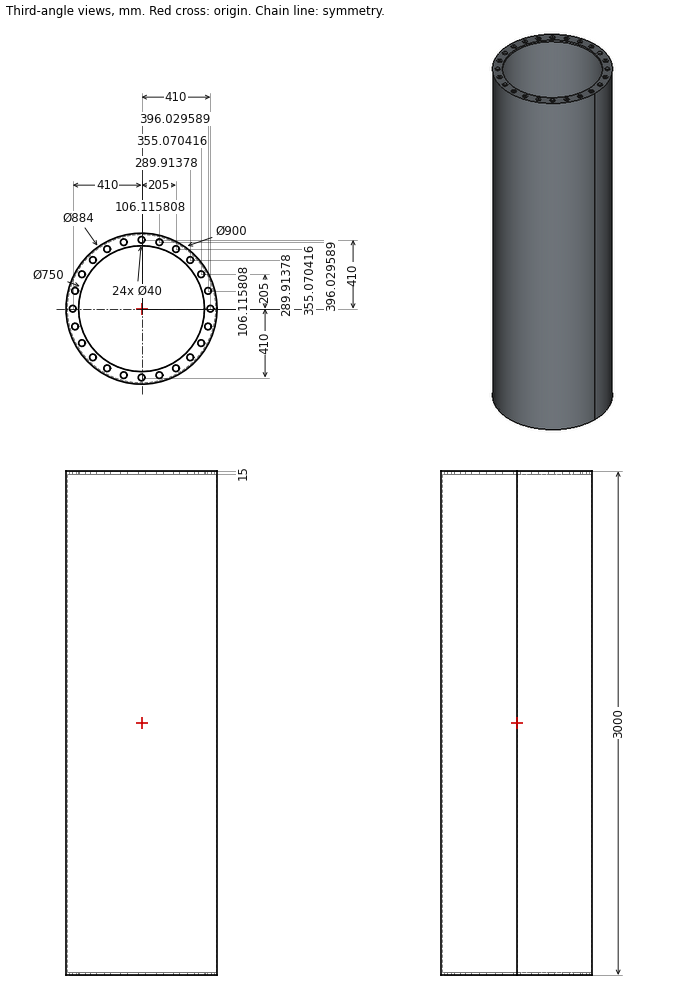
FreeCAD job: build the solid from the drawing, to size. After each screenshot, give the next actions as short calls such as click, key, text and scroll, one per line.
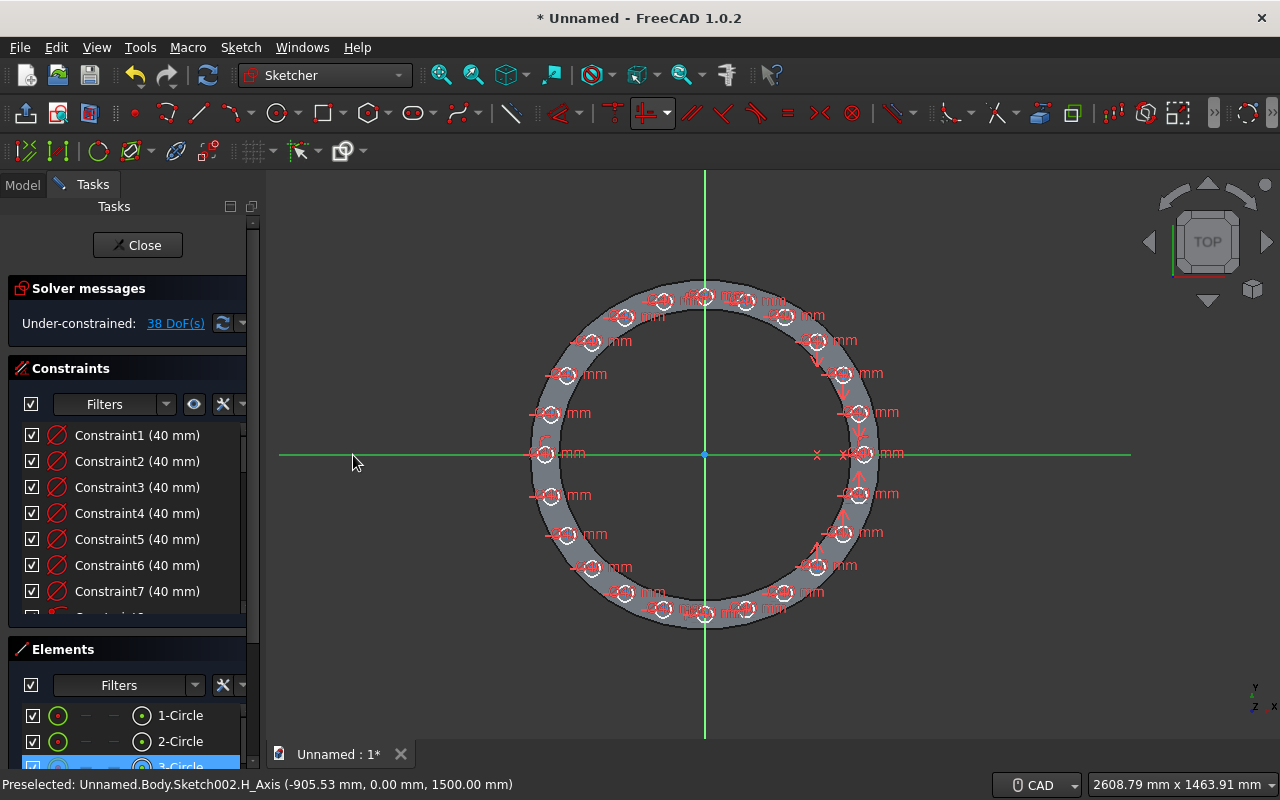
click(820, 114)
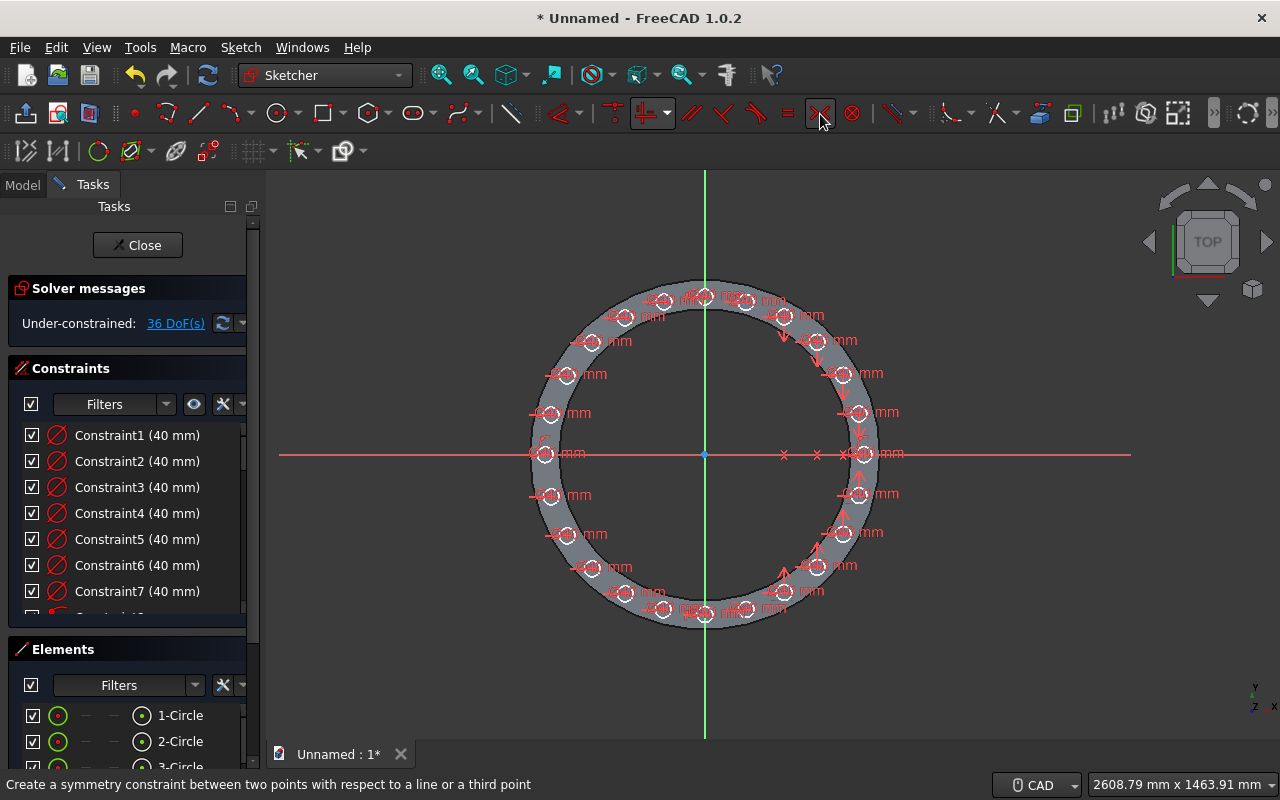
click(746, 302)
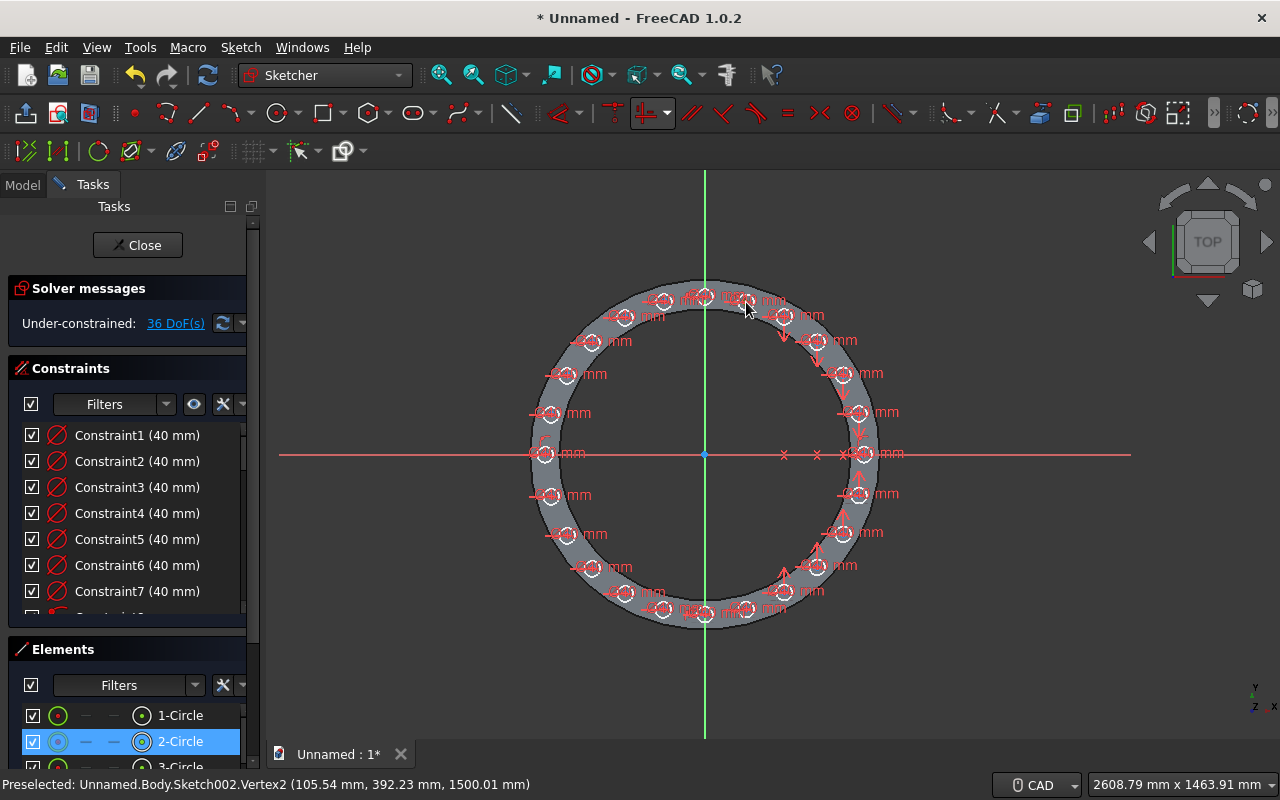
click(746, 610)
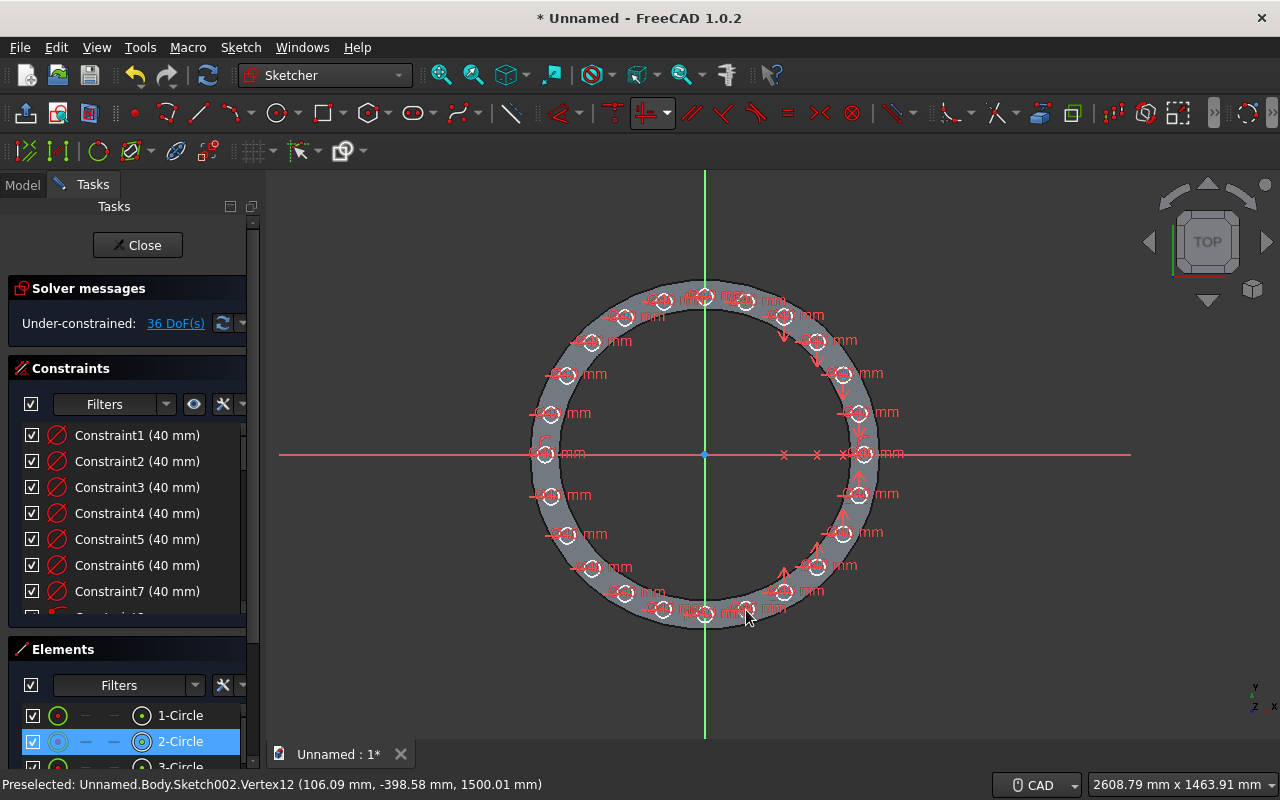
click(353, 455)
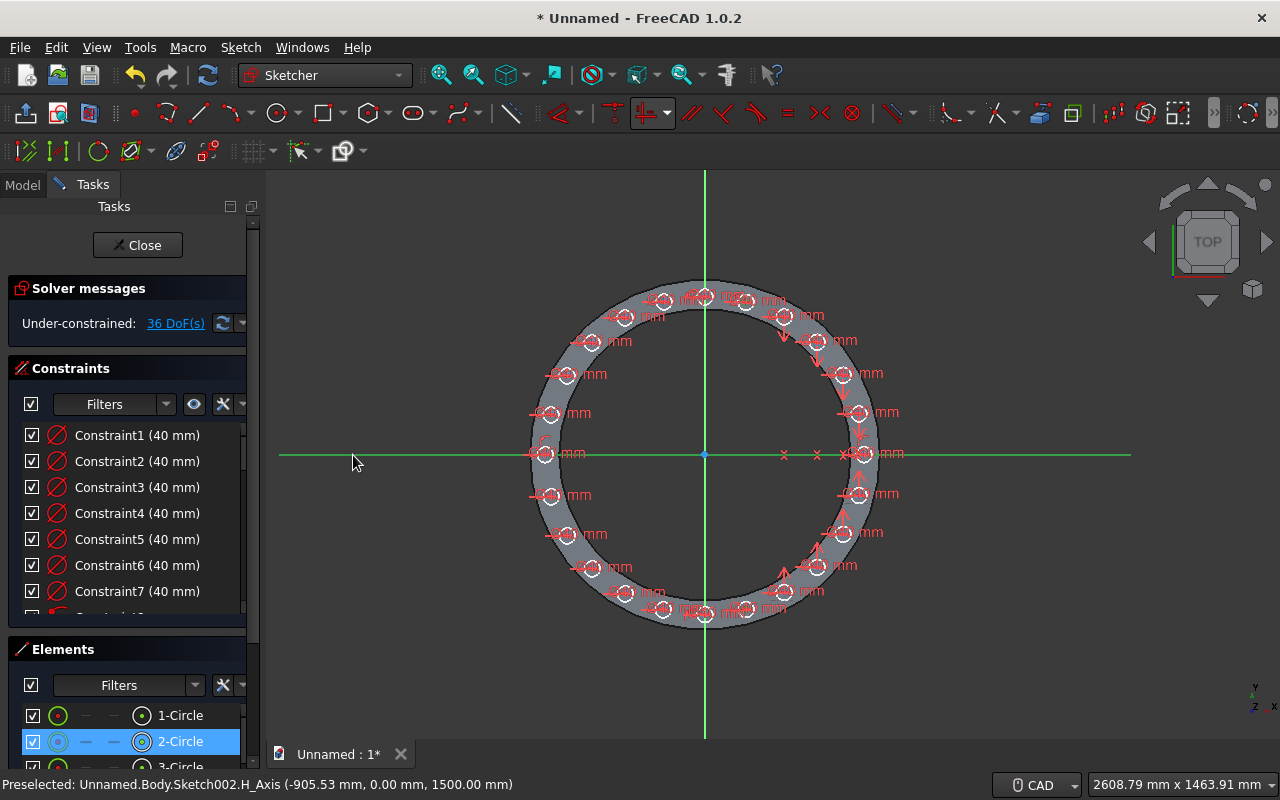
click(820, 114)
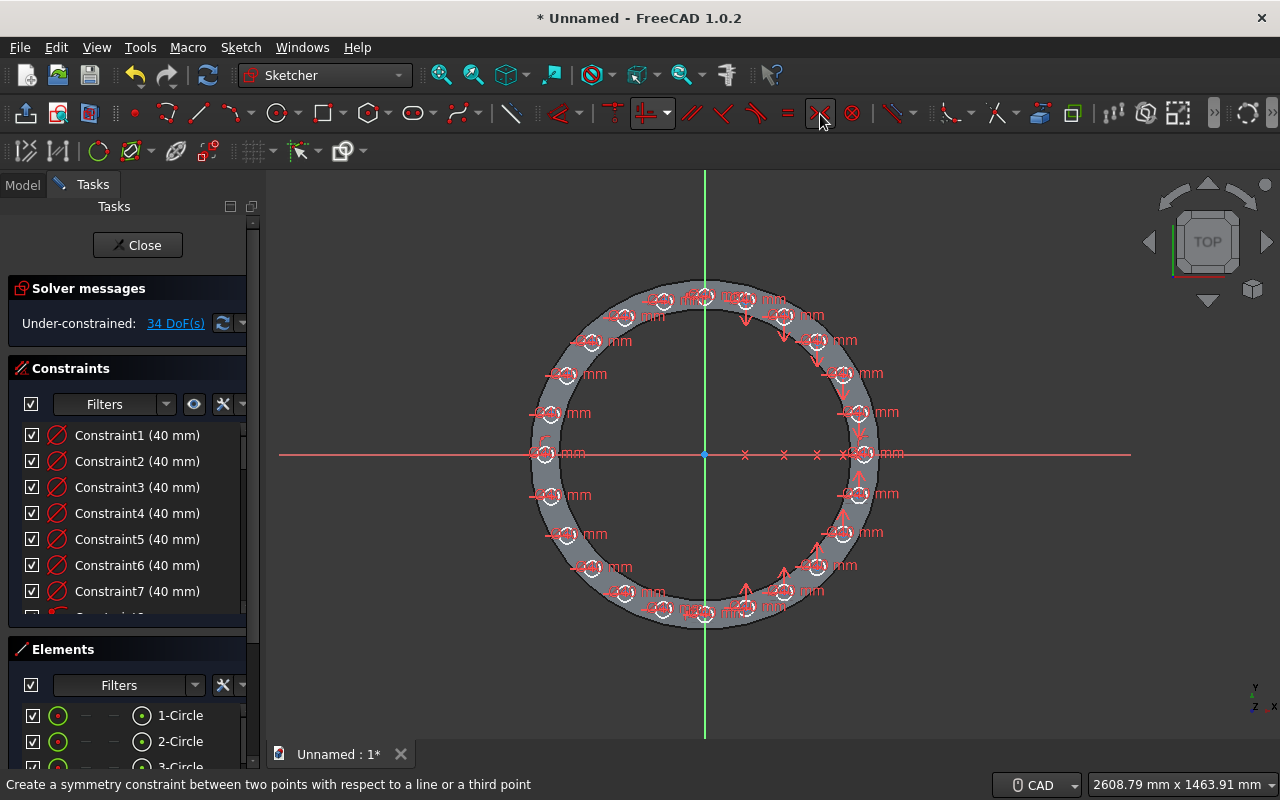
click(746, 608)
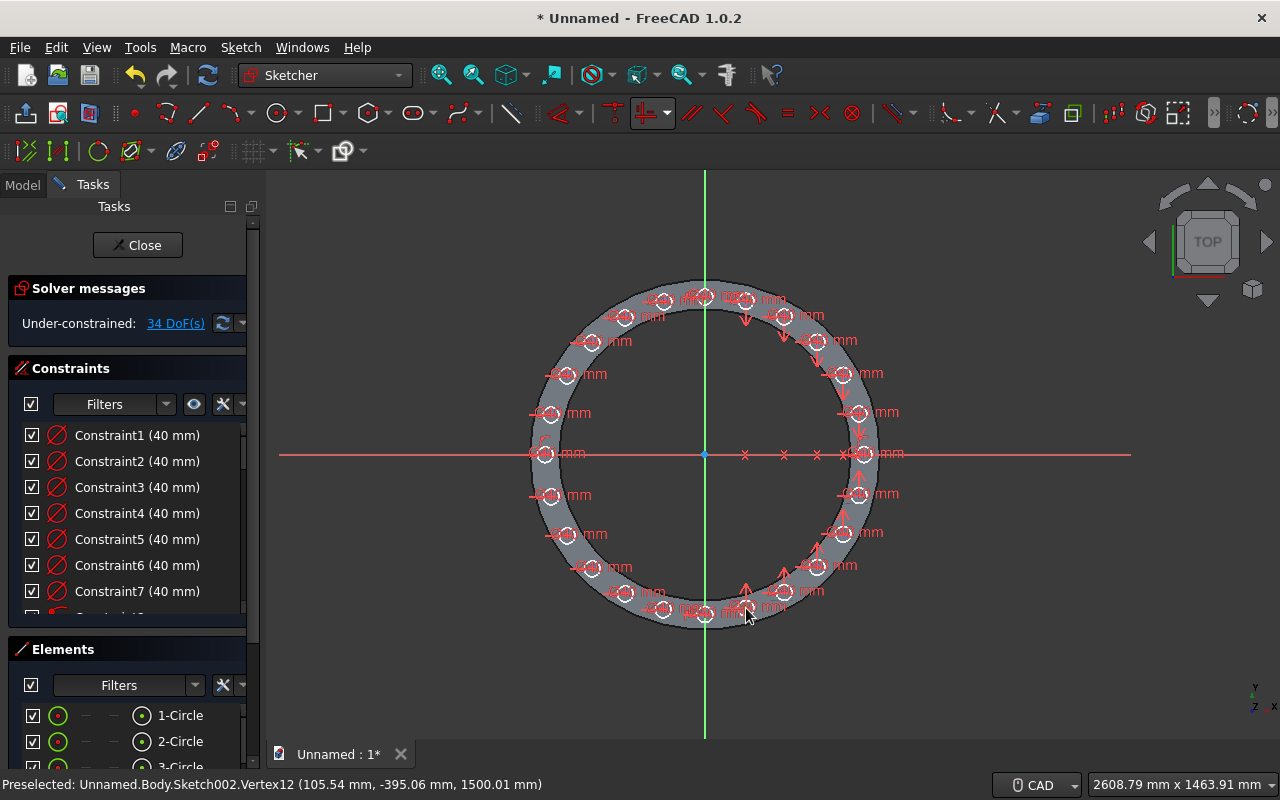
click(663, 610)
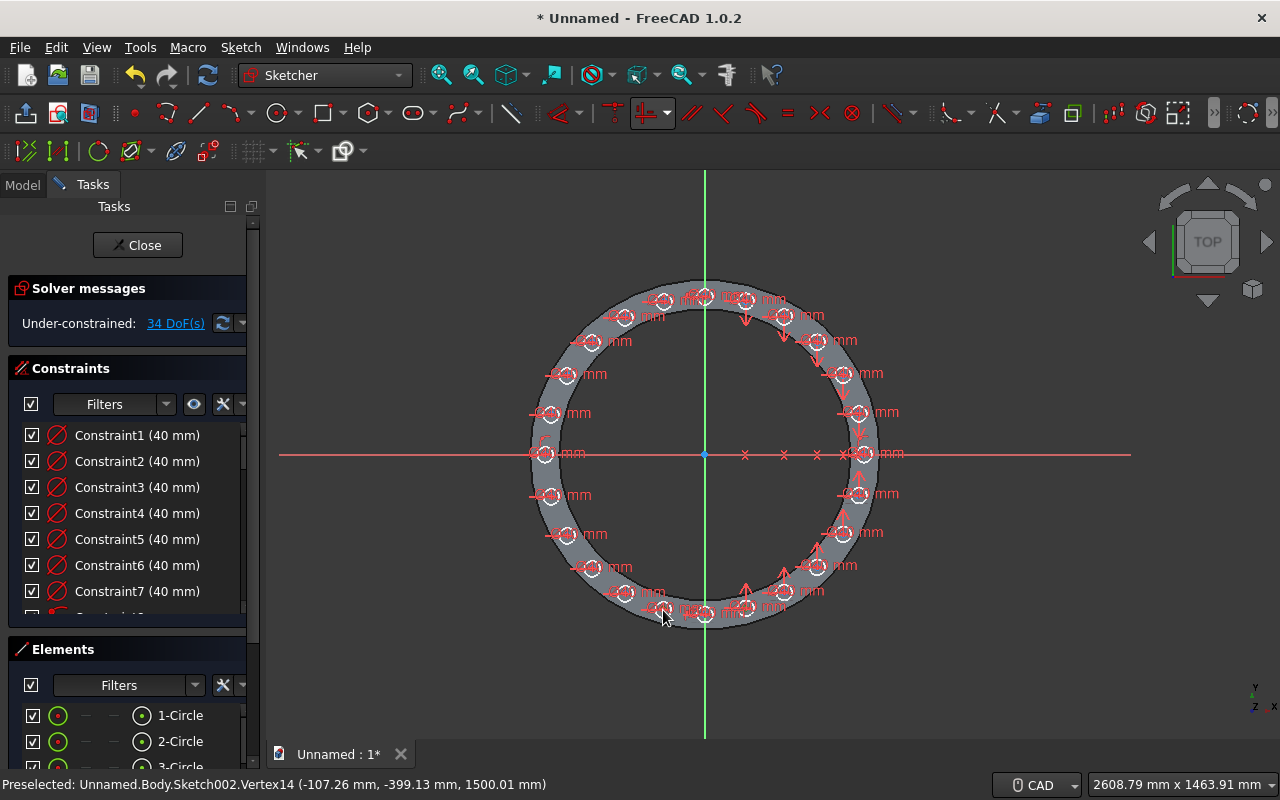
click(705, 674)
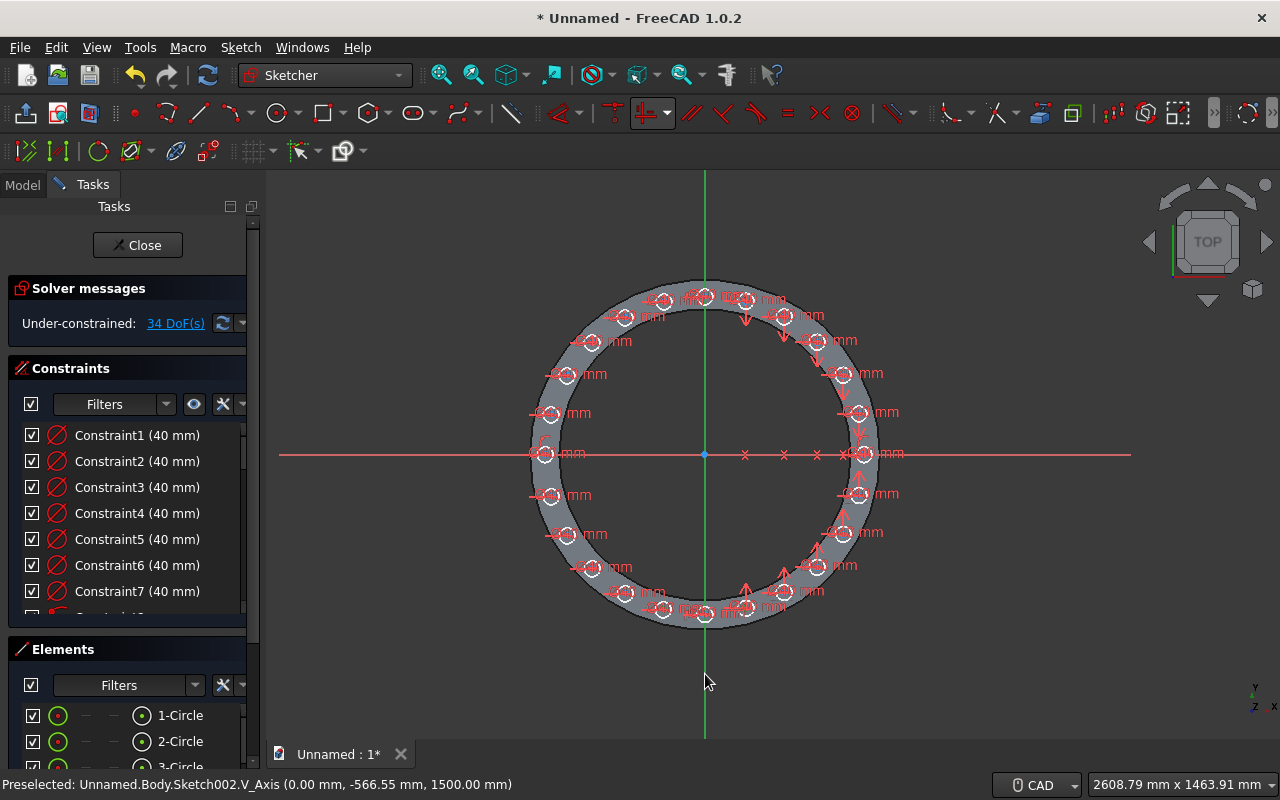
click(820, 114)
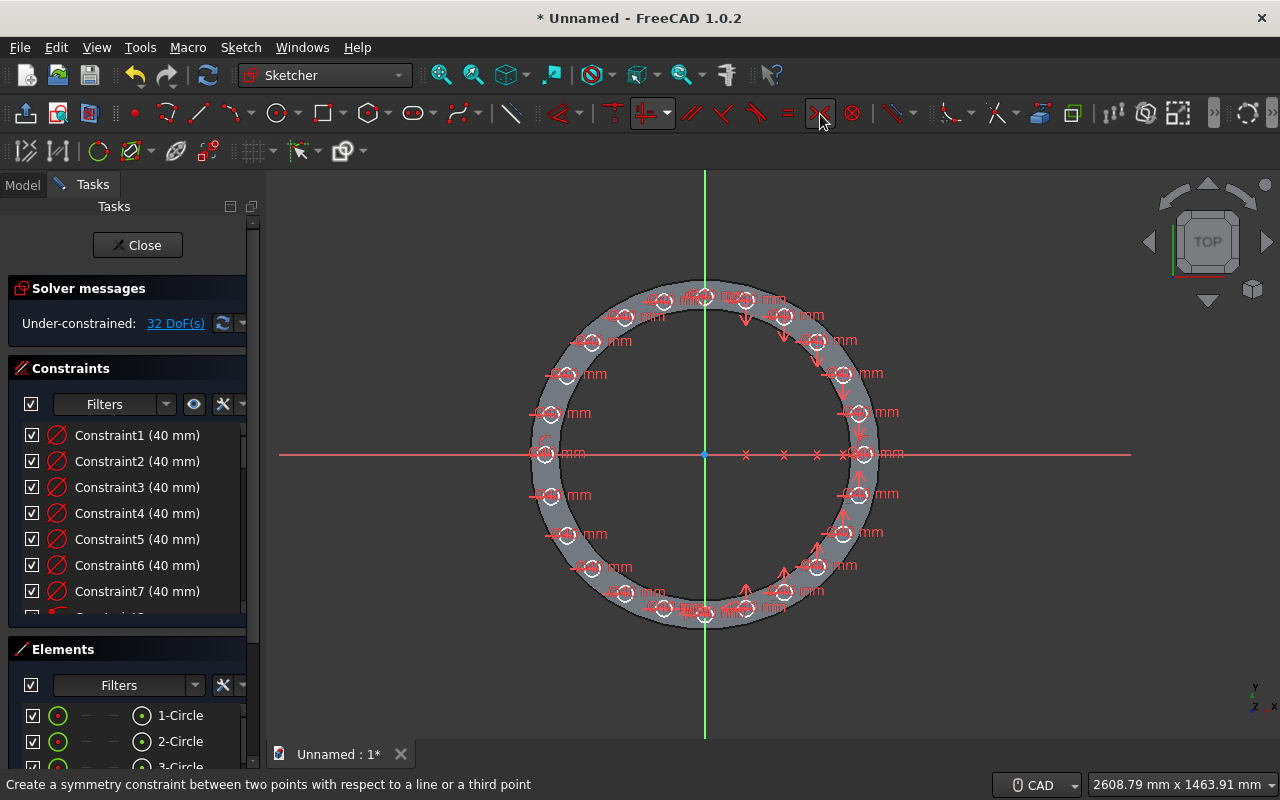
click(784, 593)